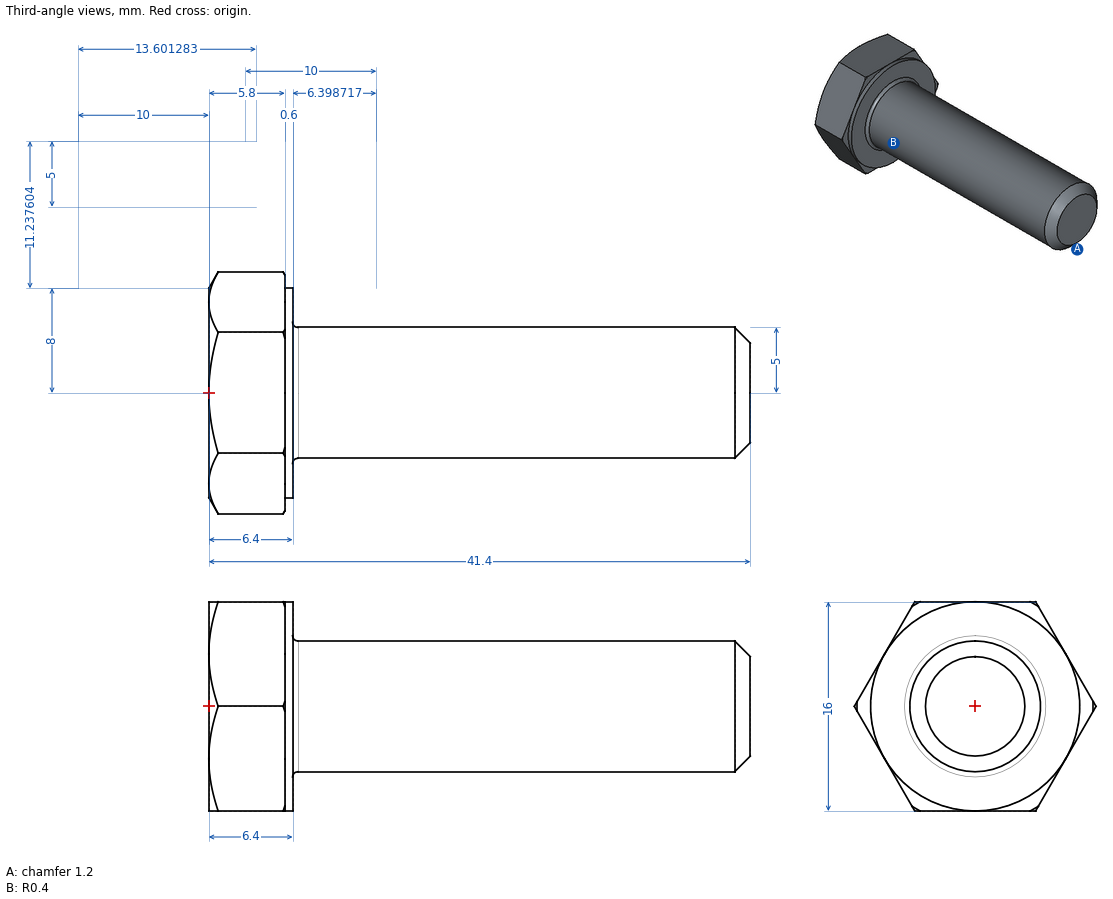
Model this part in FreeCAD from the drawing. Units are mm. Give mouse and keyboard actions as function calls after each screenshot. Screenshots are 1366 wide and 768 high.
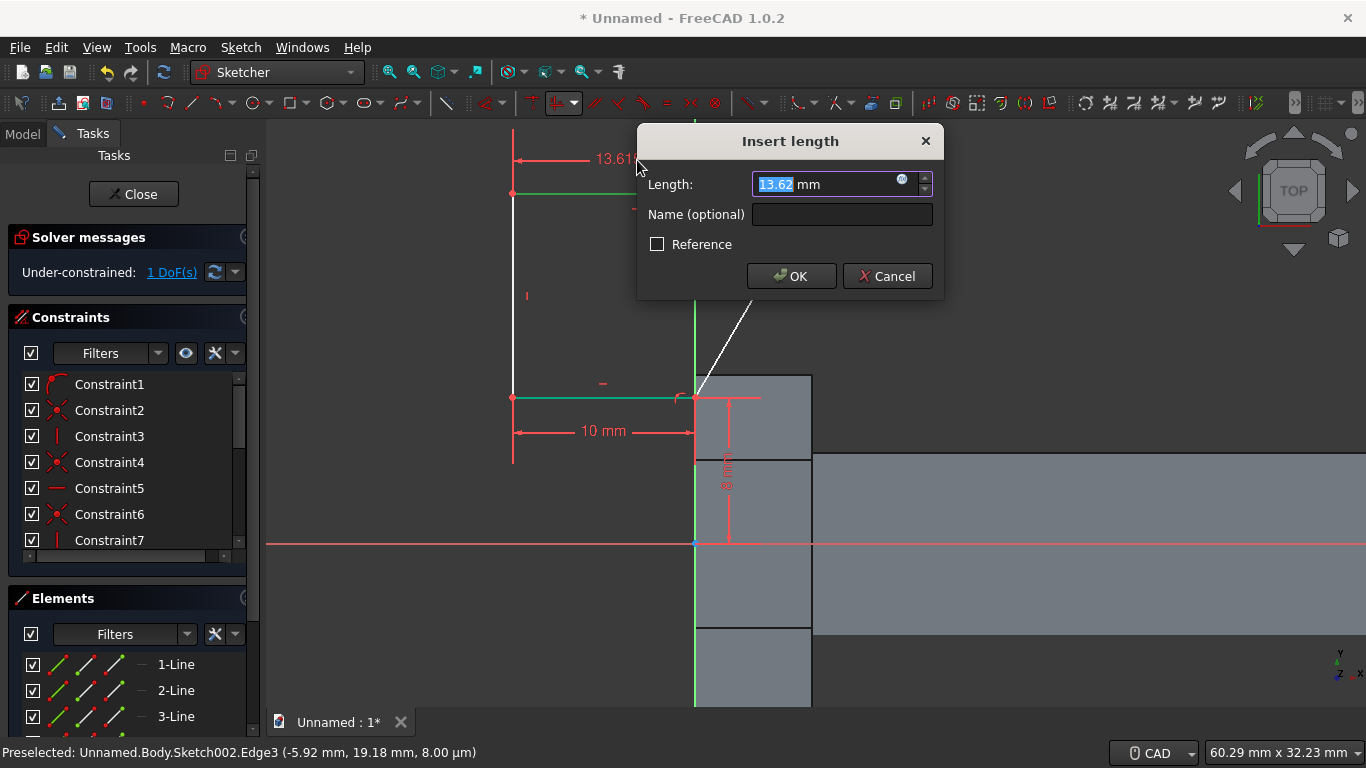
text(13.601283)
key(Return)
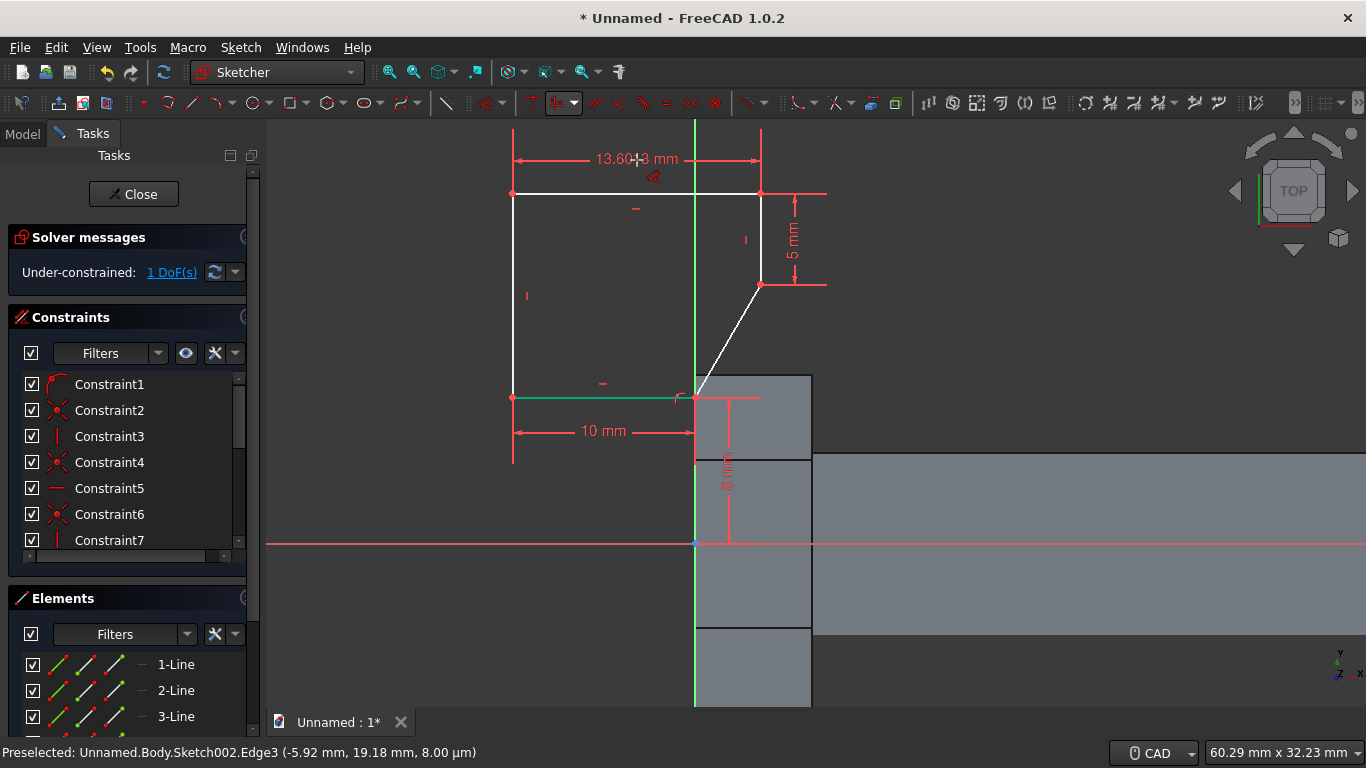
click(513, 255)
click(479, 296)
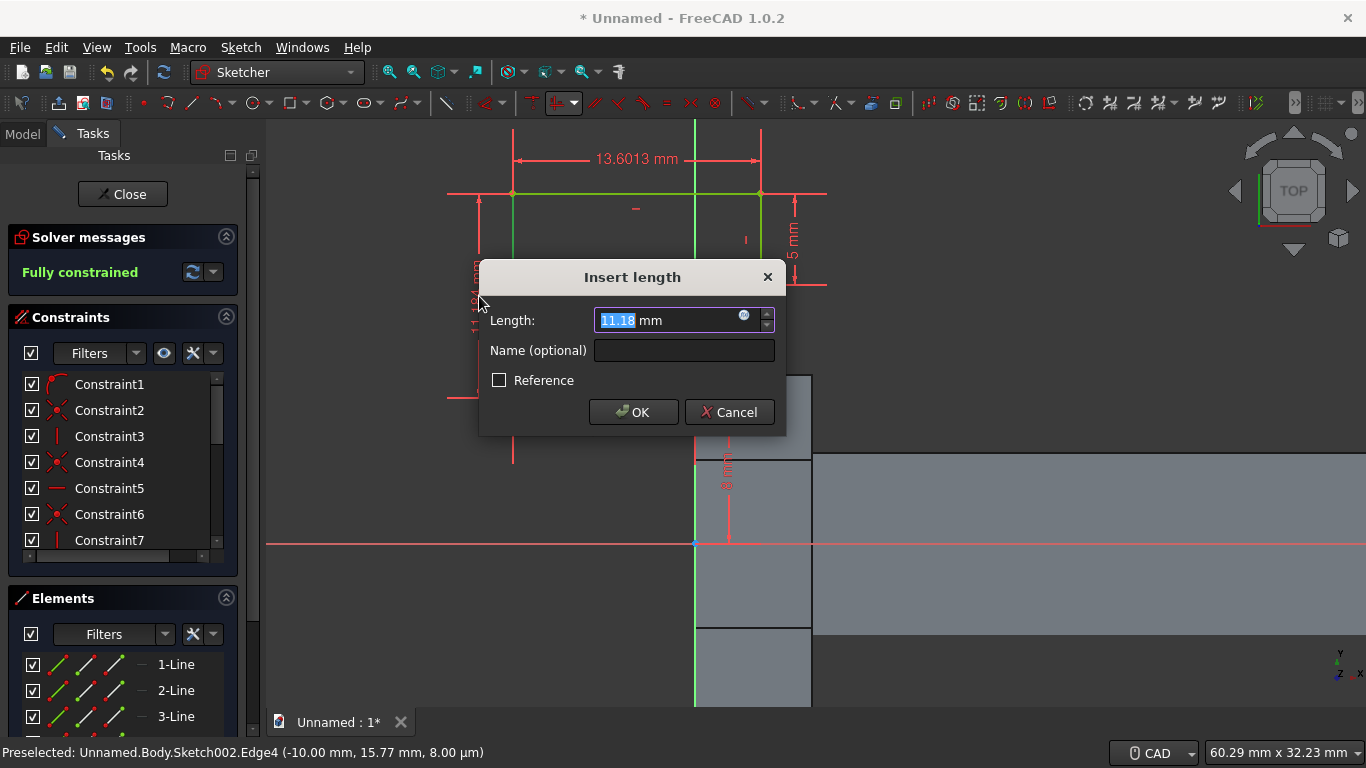
text(11.237604)
key(Return)
key(Escape)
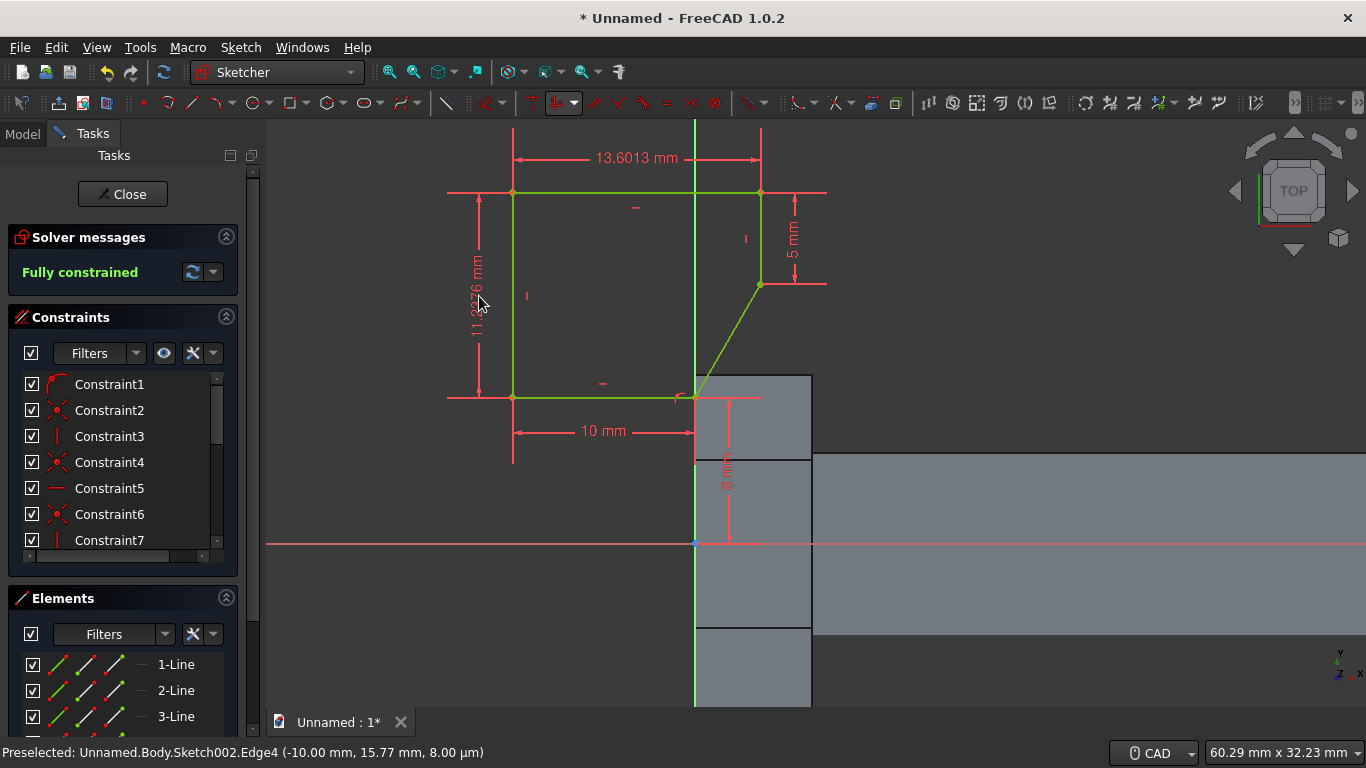
click(123, 194)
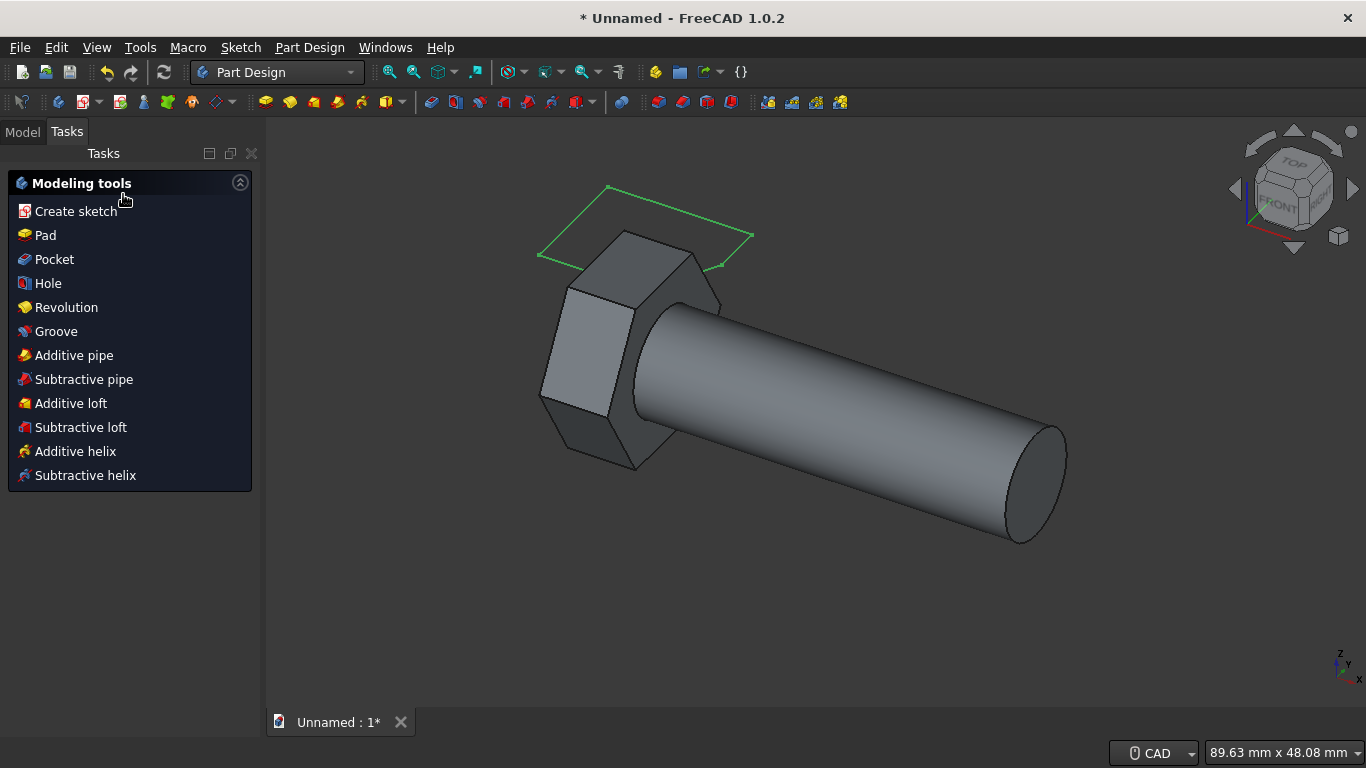
click(480, 102)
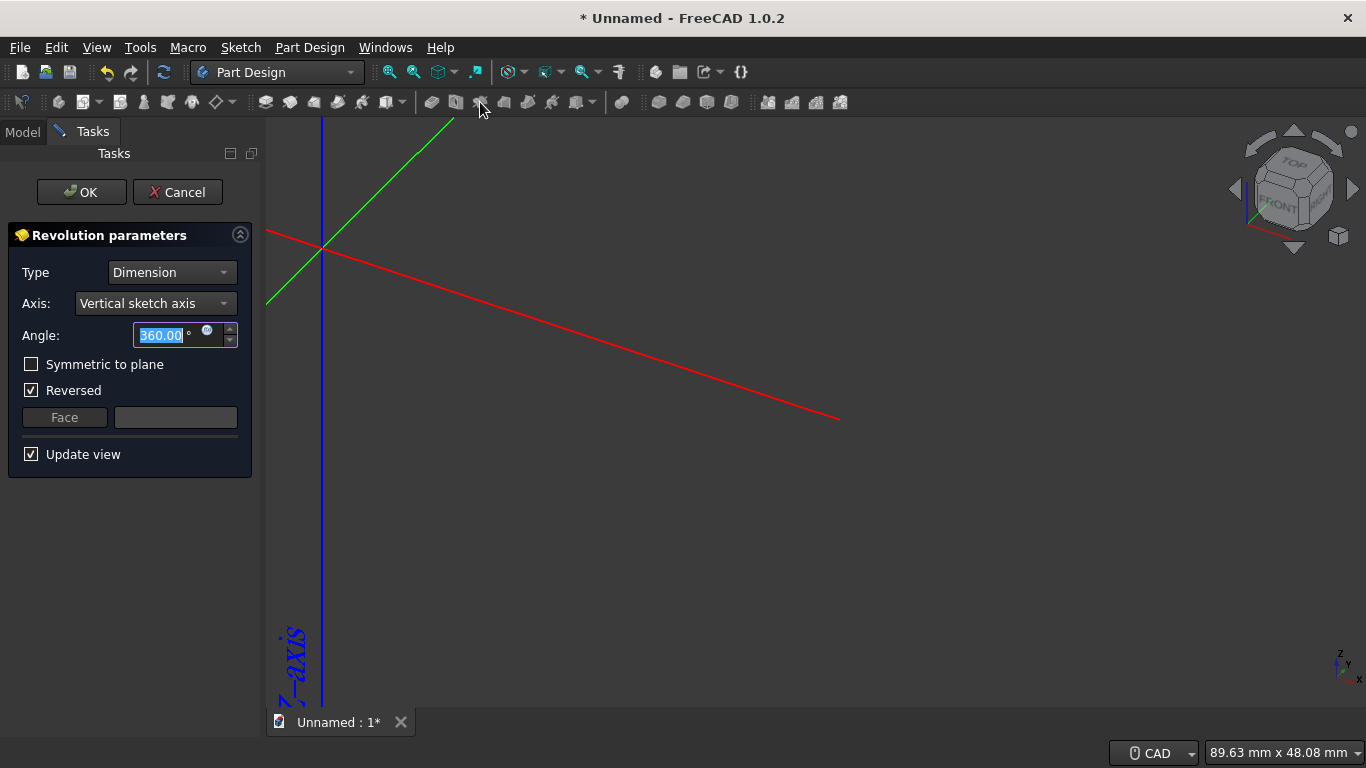
click(156, 304)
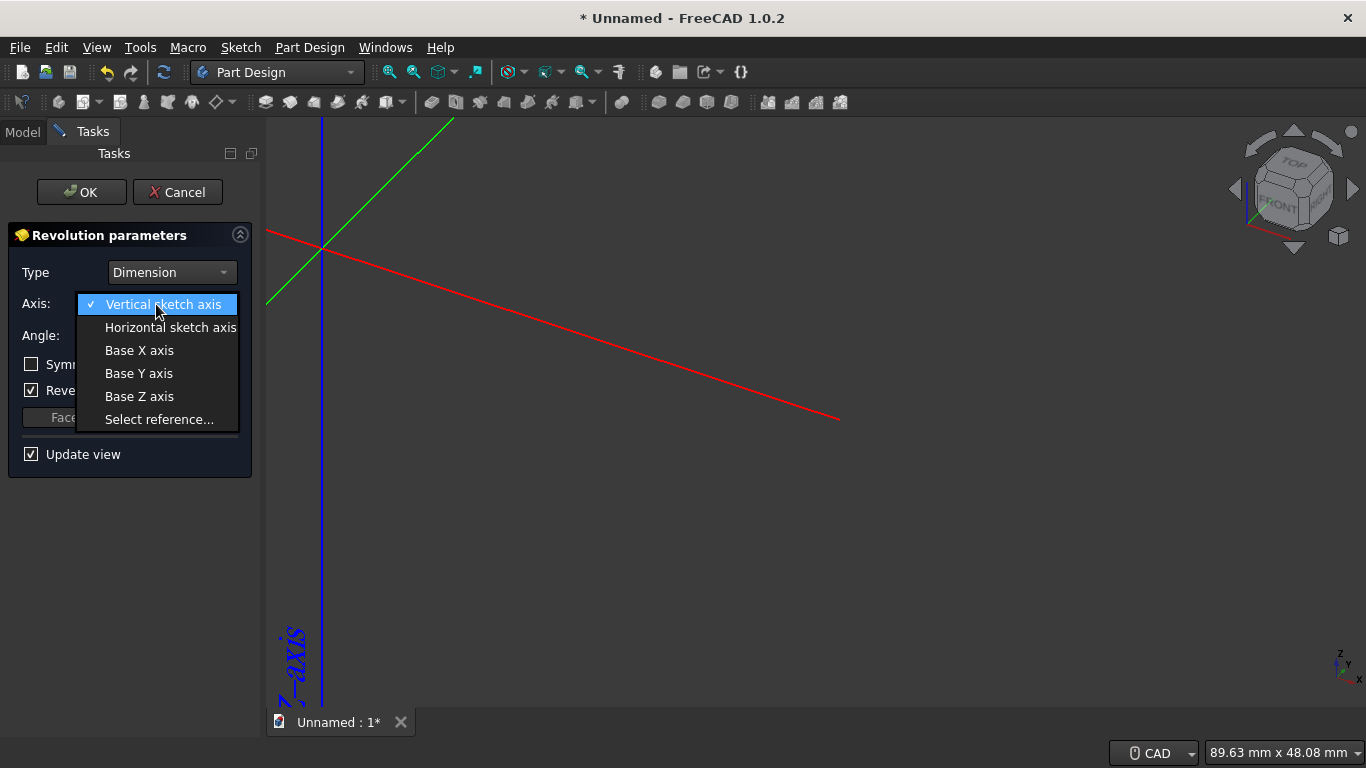
click(156, 328)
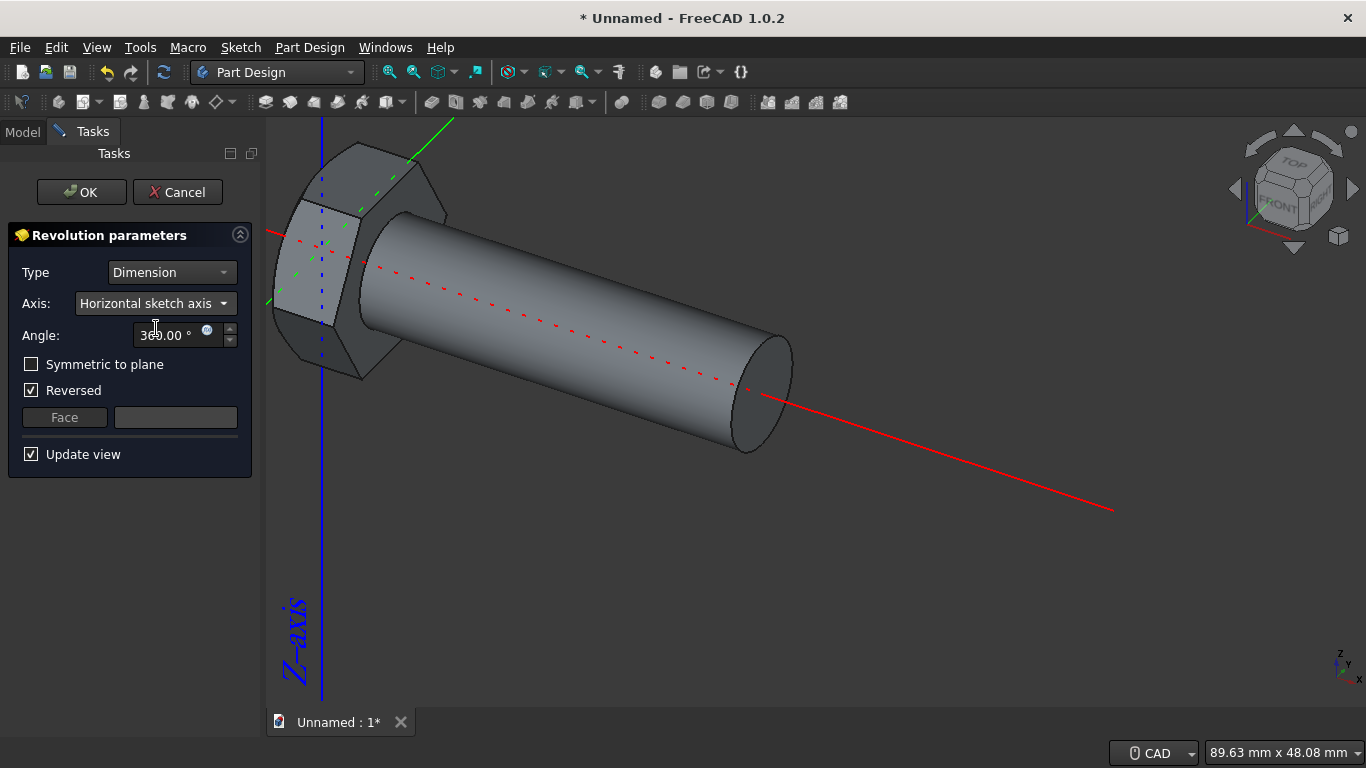
click(82, 192)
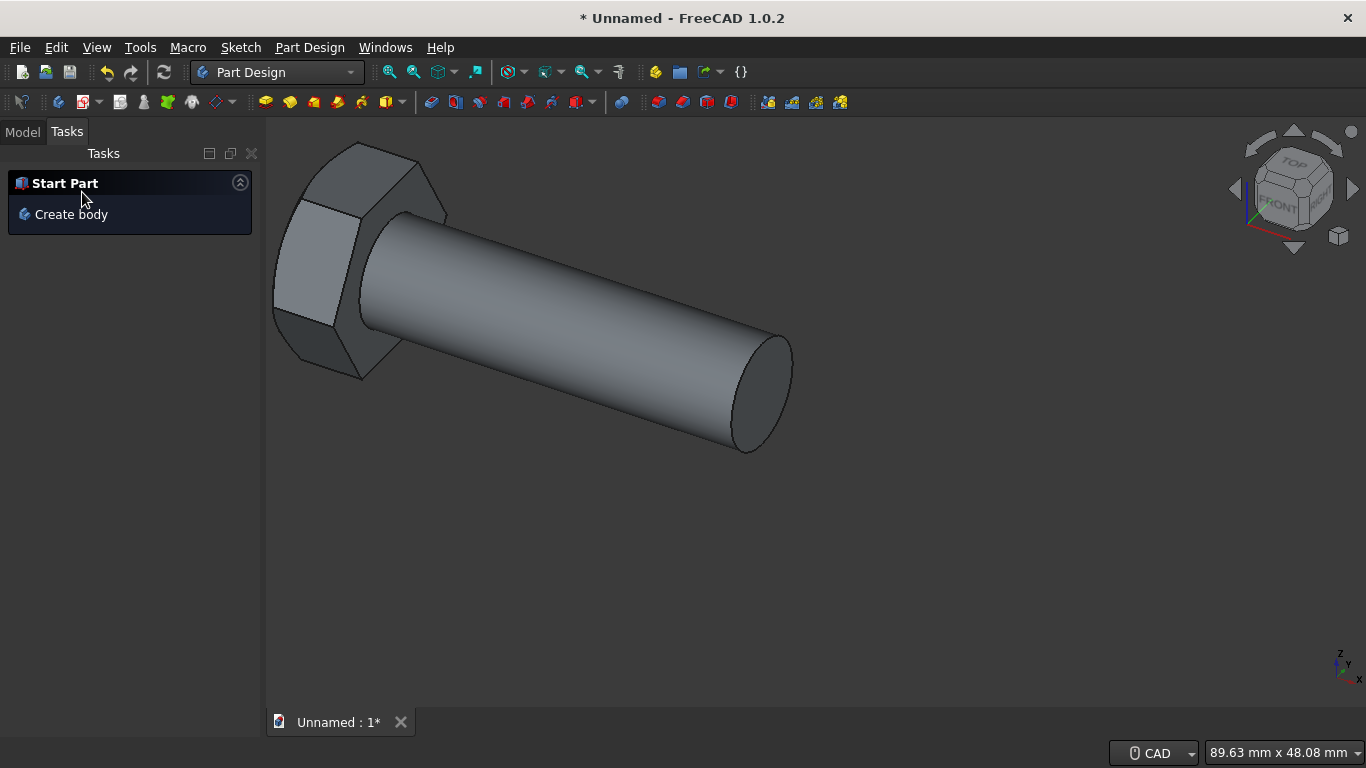
click(390, 72)